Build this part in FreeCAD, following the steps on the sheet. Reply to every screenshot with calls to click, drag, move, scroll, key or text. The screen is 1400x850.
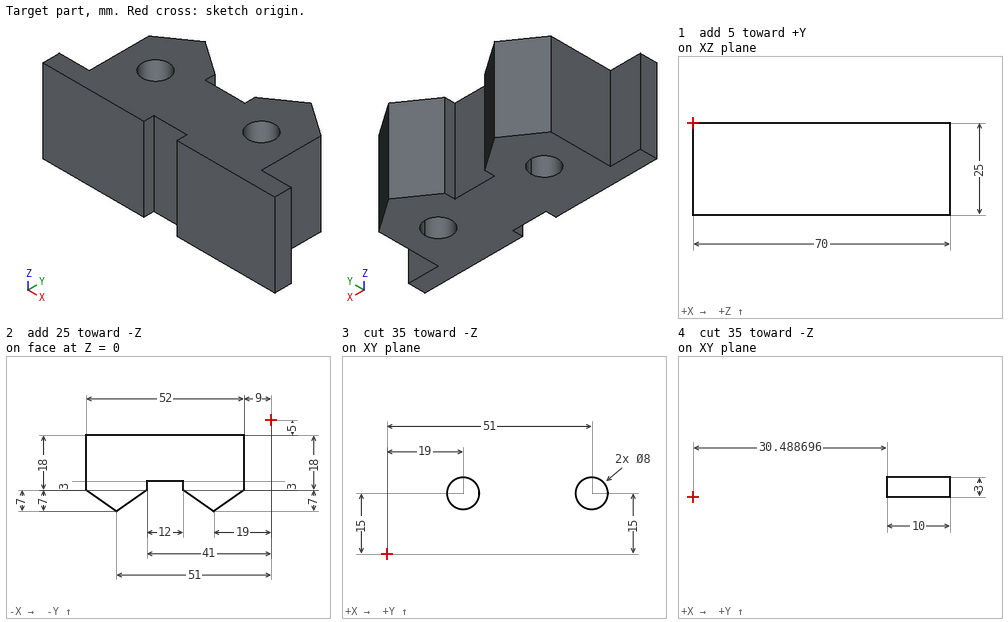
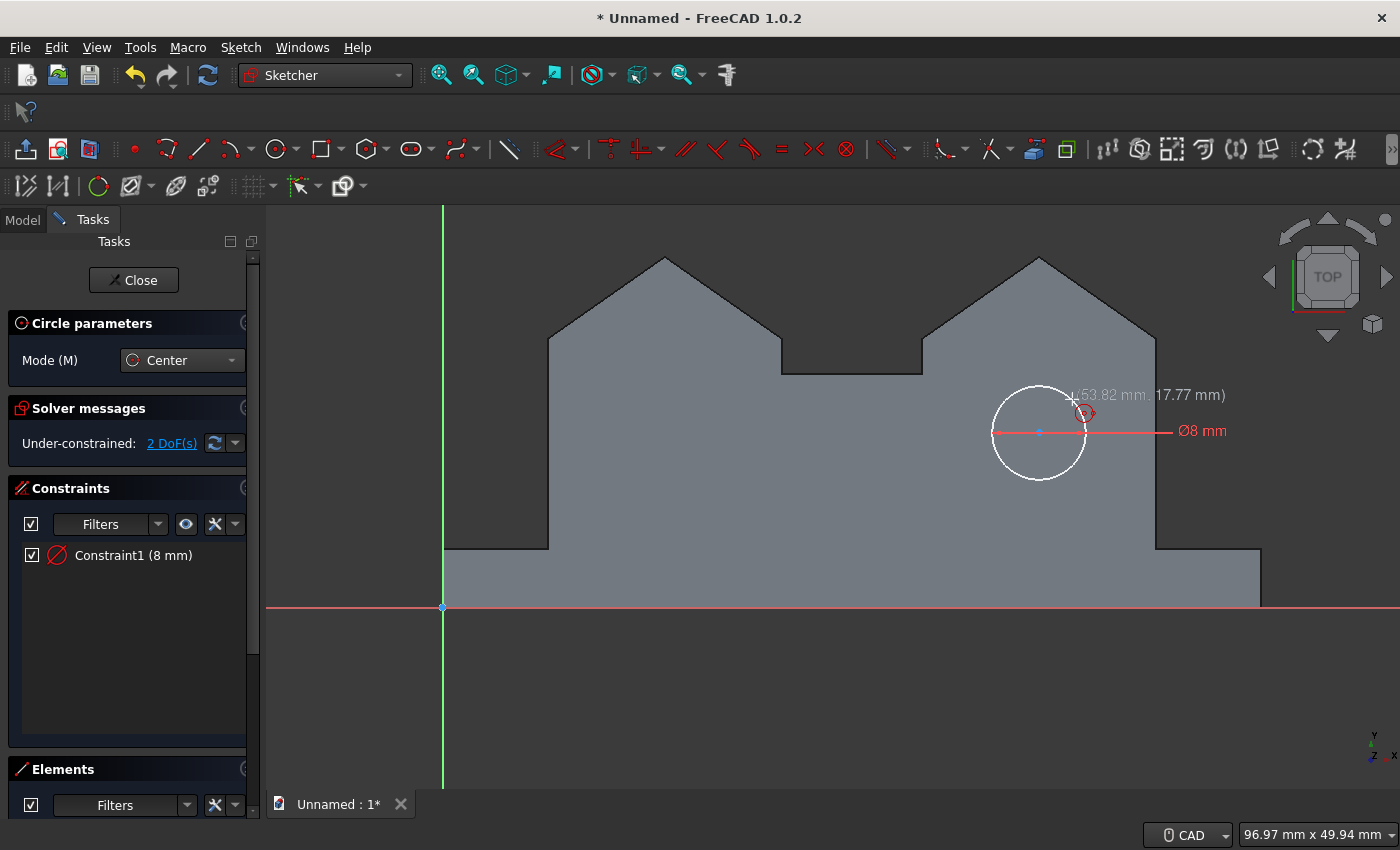
click(665, 432)
move(698, 399)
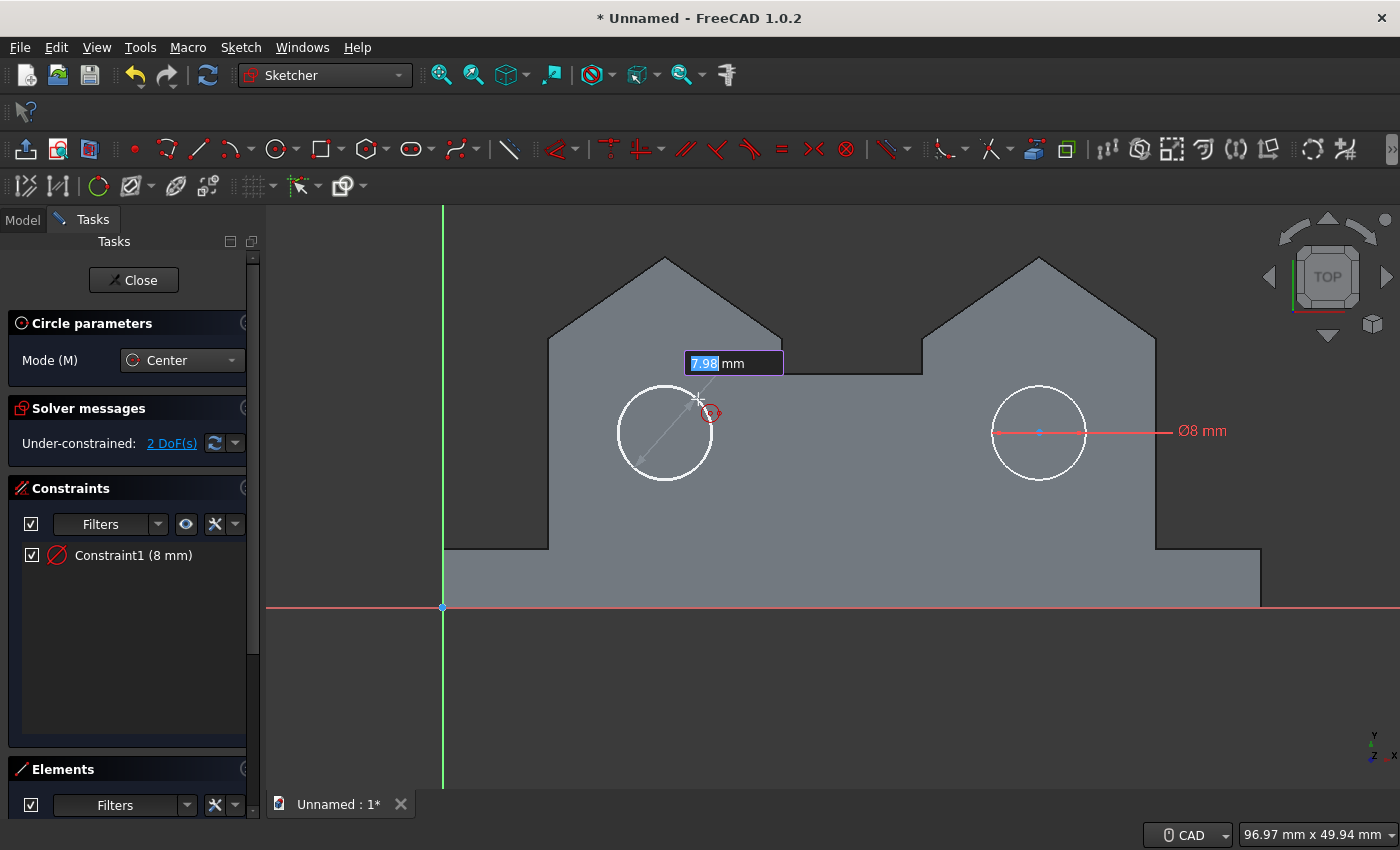
text(8)
key(Return)
key(Escape)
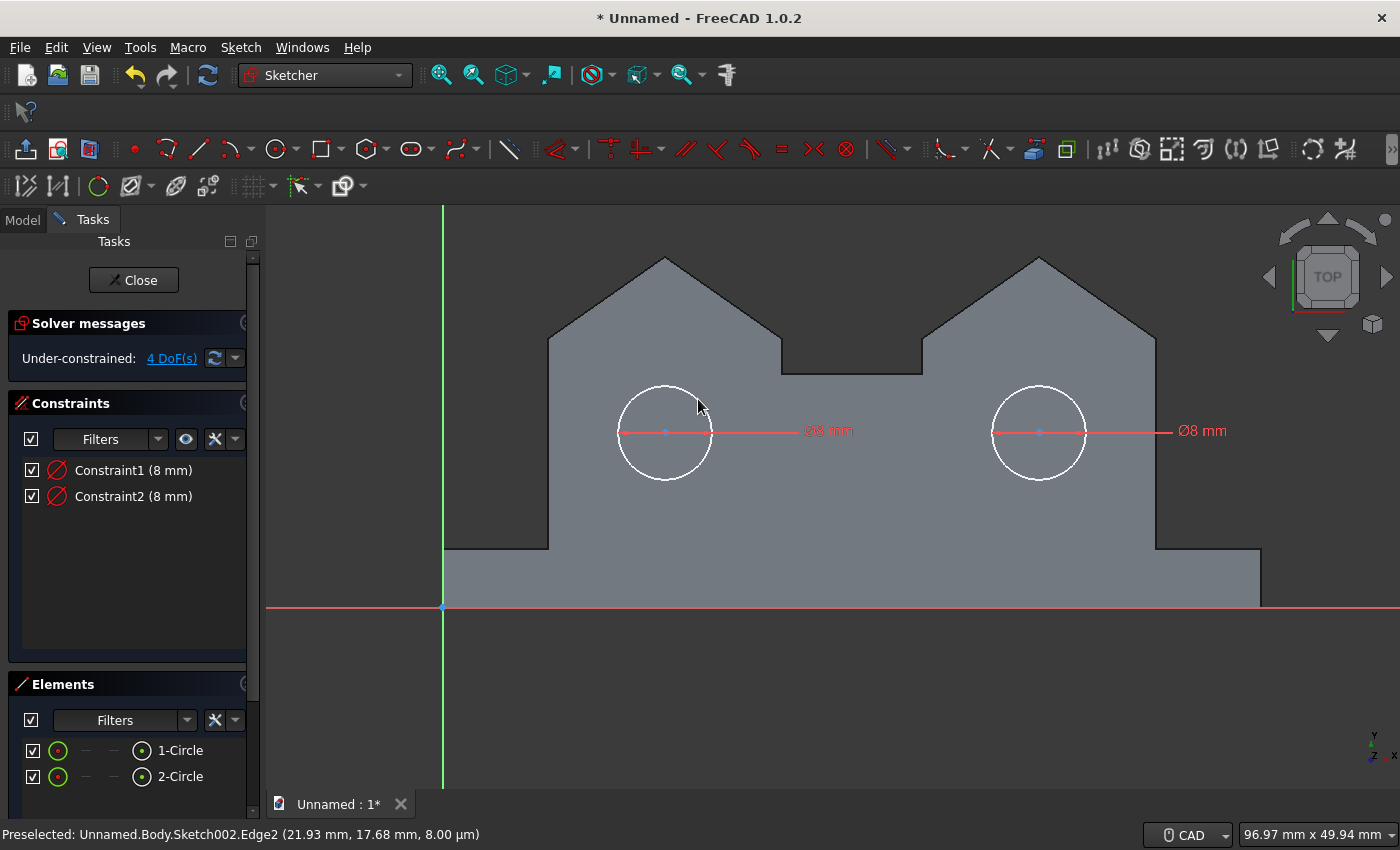
key(d)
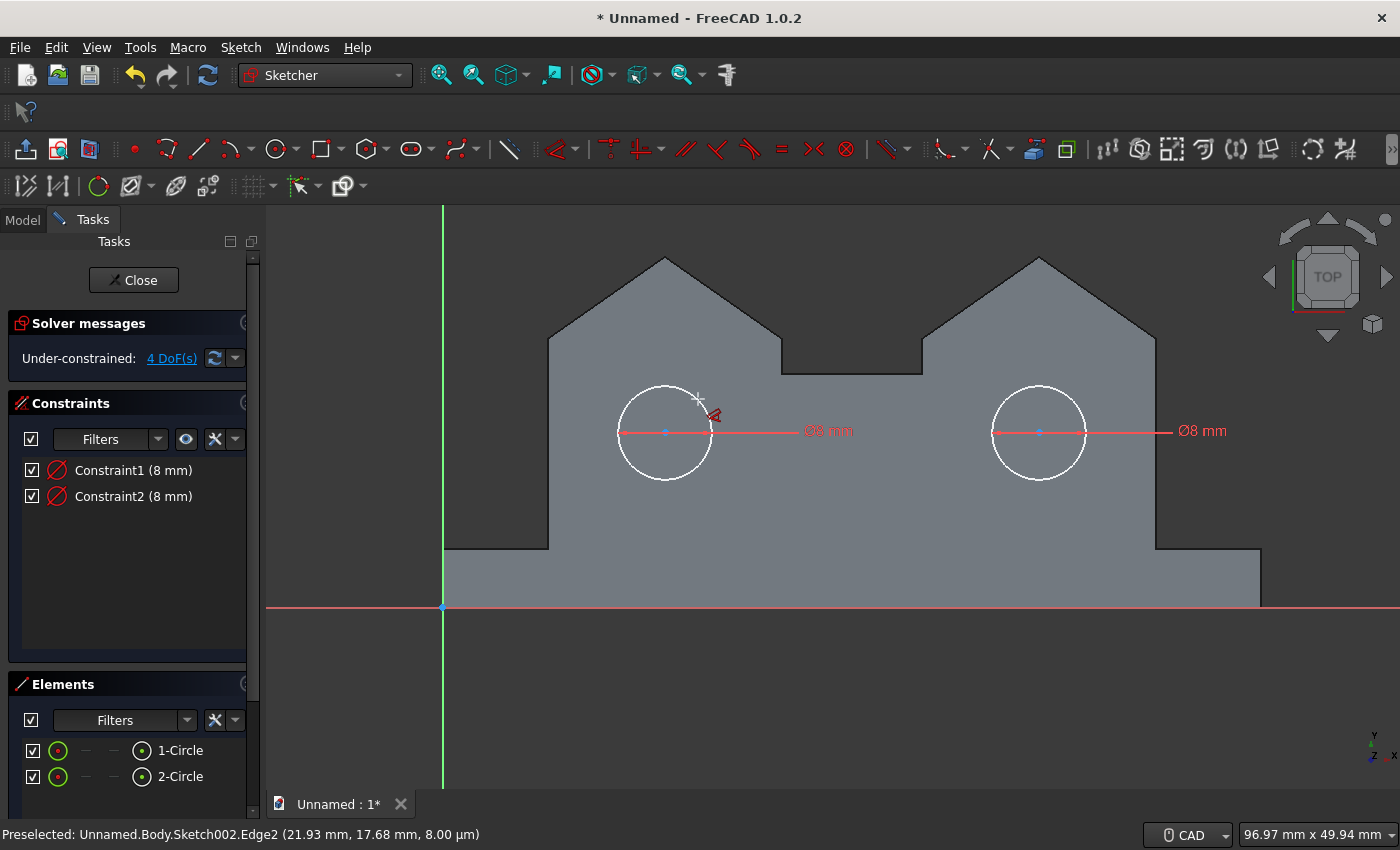
click(1039, 433)
click(741, 642)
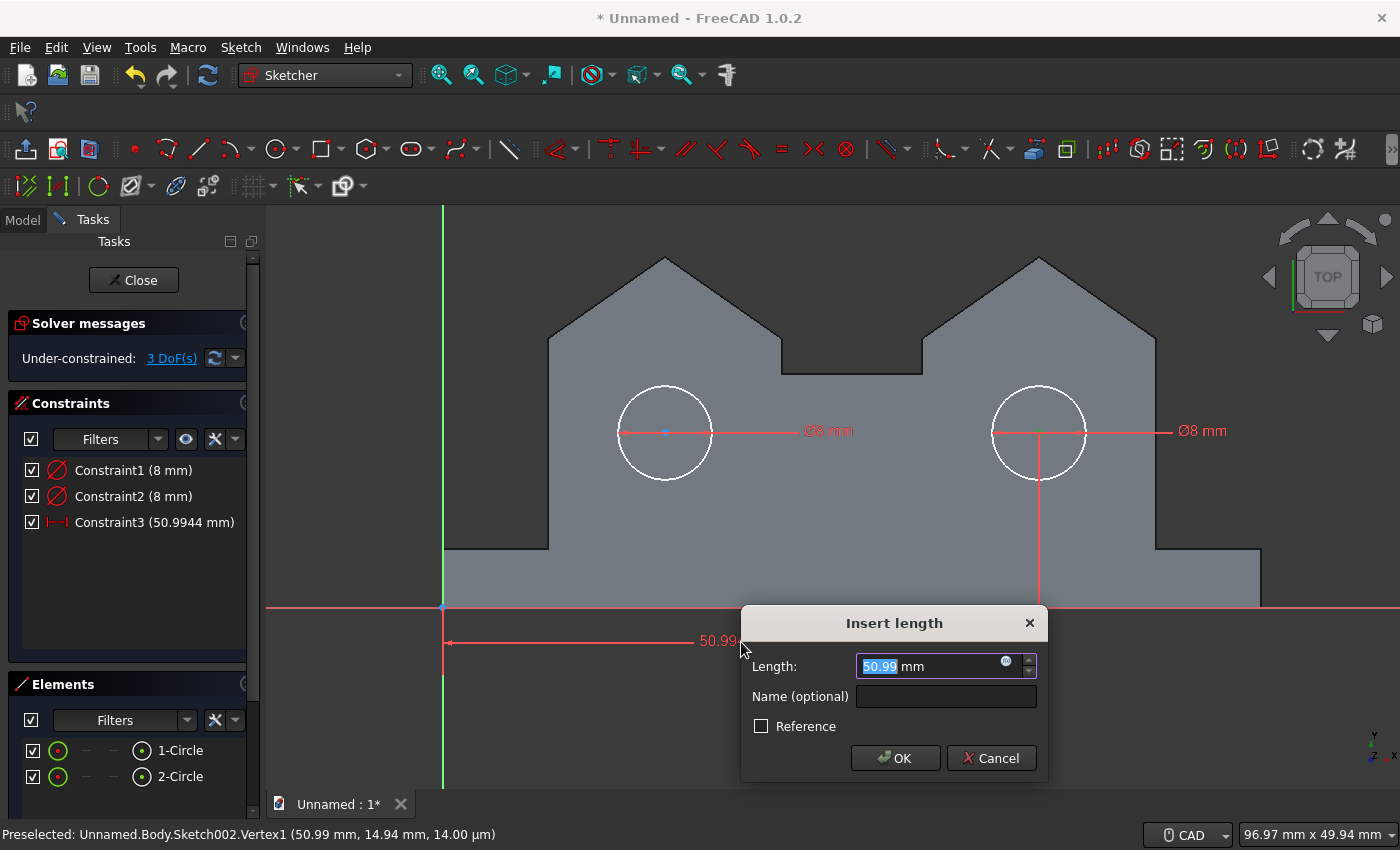
text(51)
key(Return)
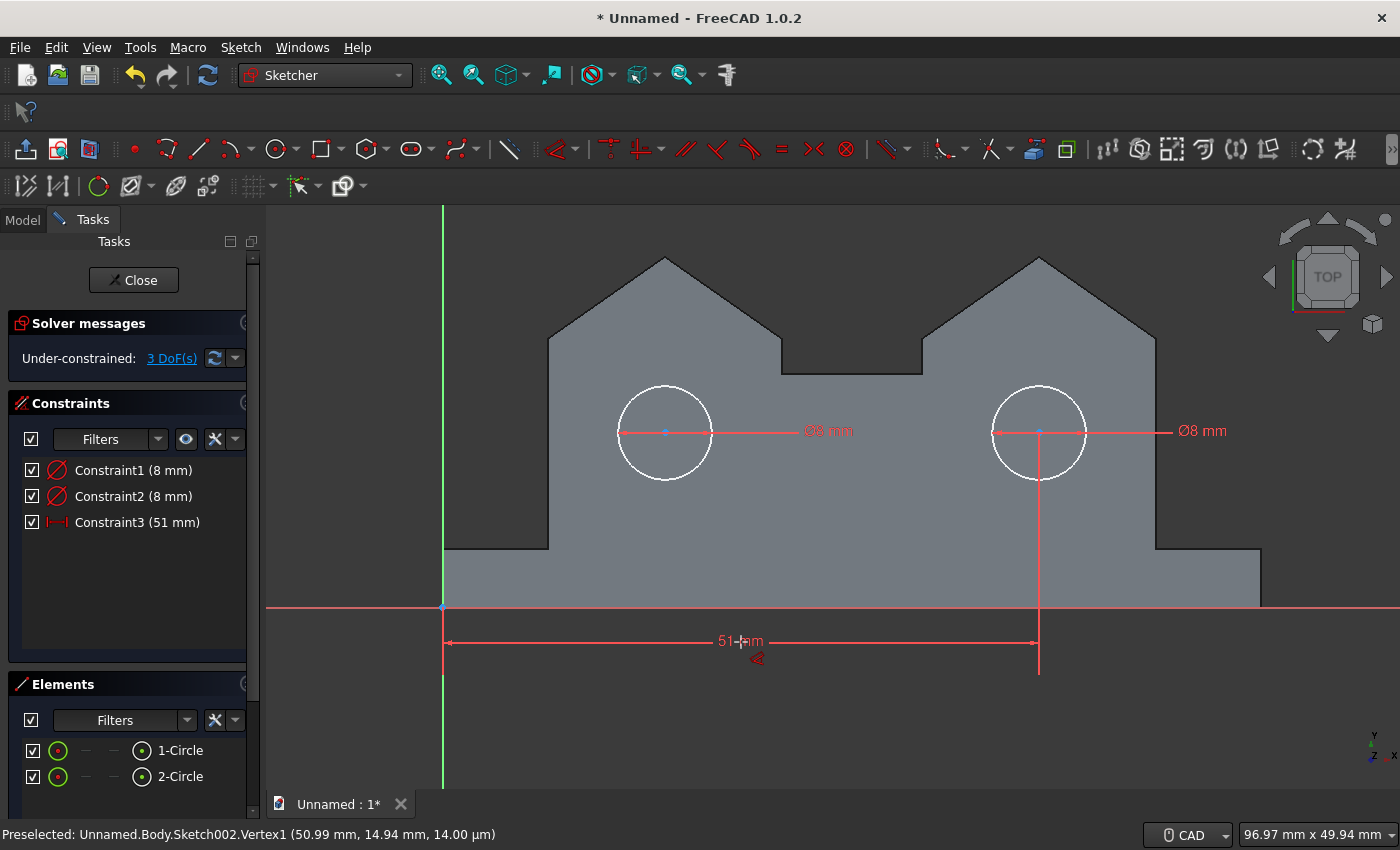
click(1039, 433)
click(409, 520)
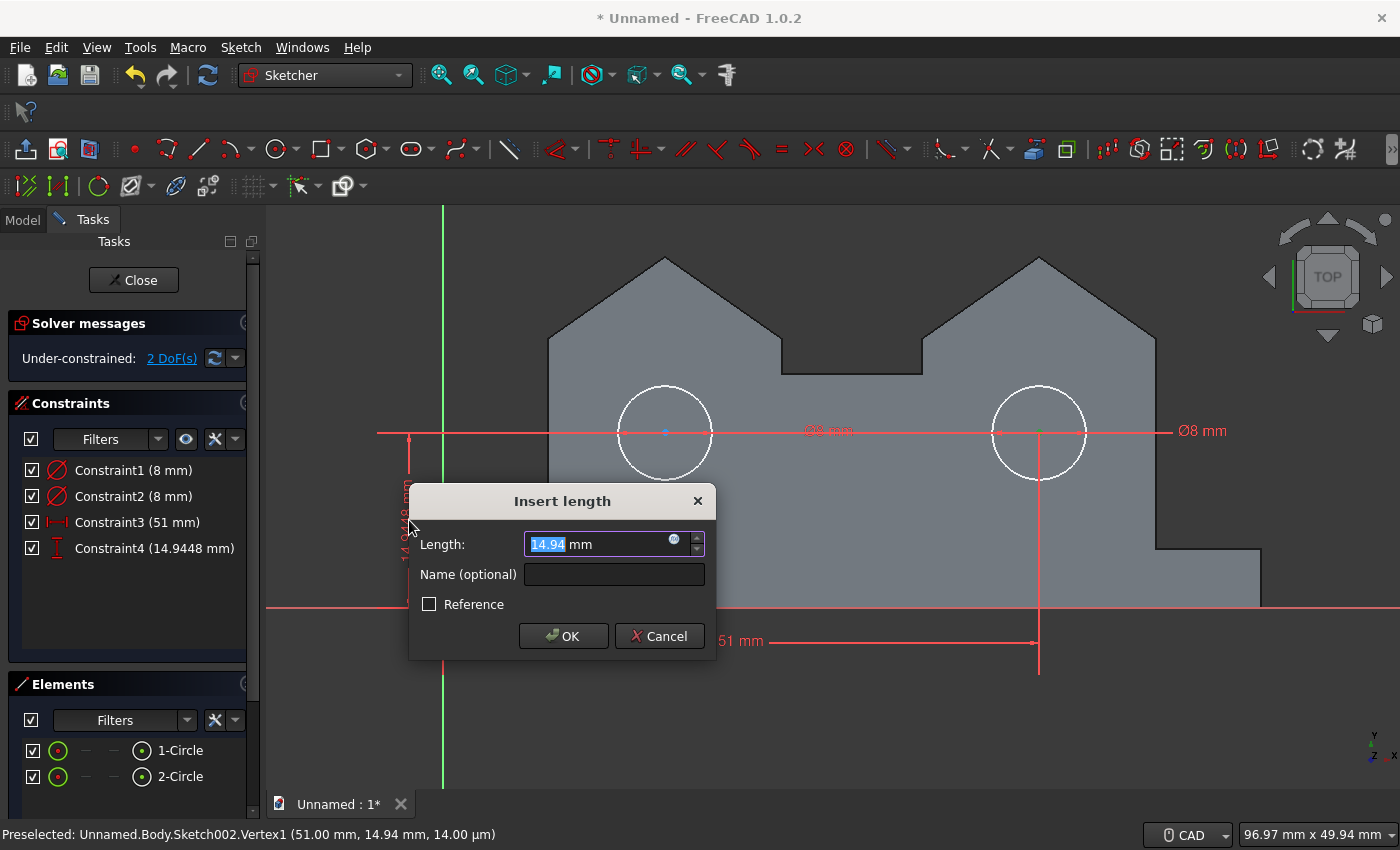
text(15)
key(Return)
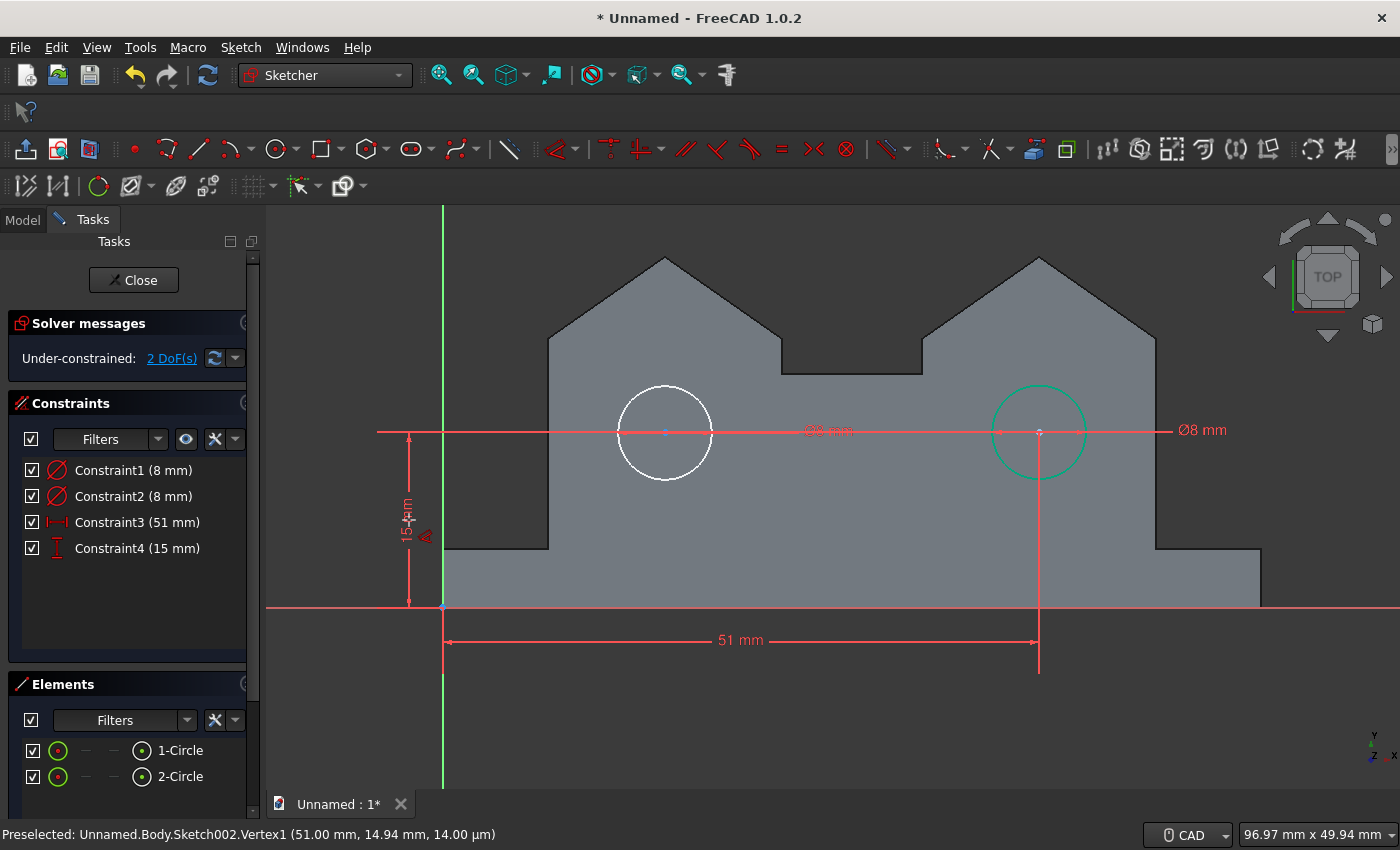
click(665, 433)
click(554, 642)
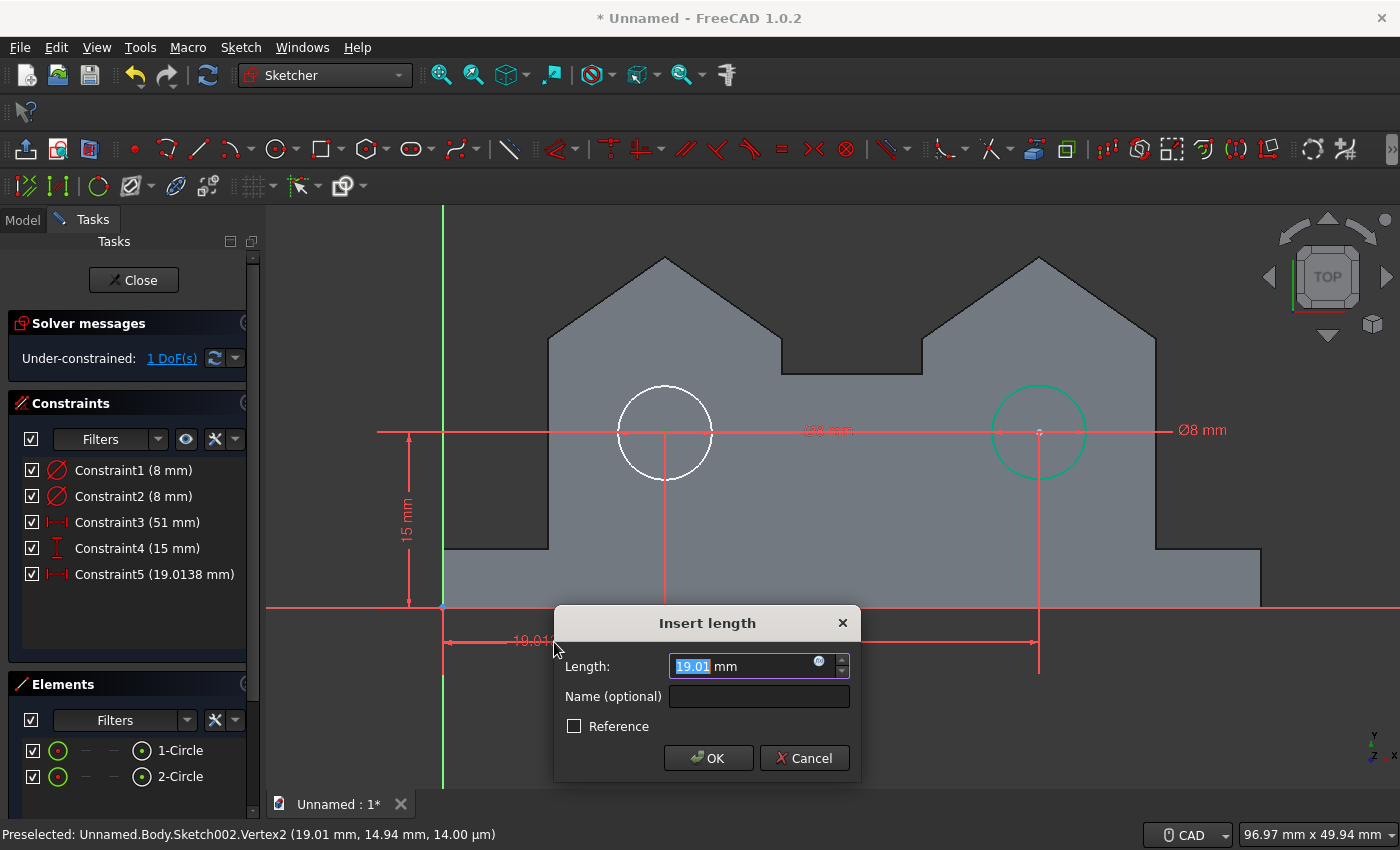
text(19)
key(Return)